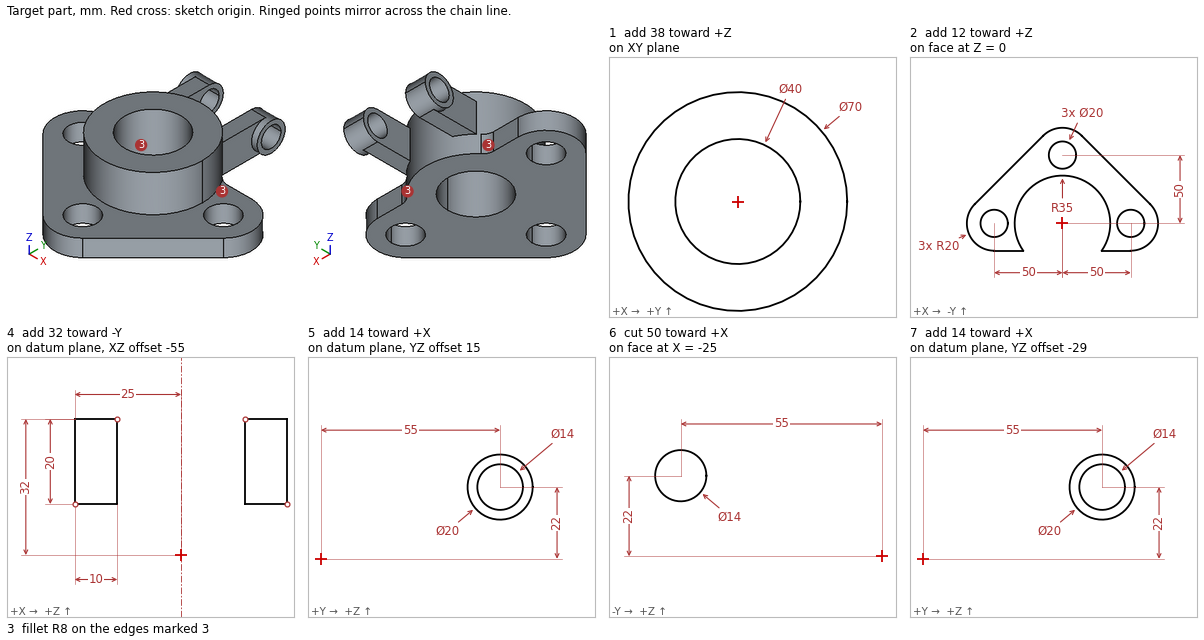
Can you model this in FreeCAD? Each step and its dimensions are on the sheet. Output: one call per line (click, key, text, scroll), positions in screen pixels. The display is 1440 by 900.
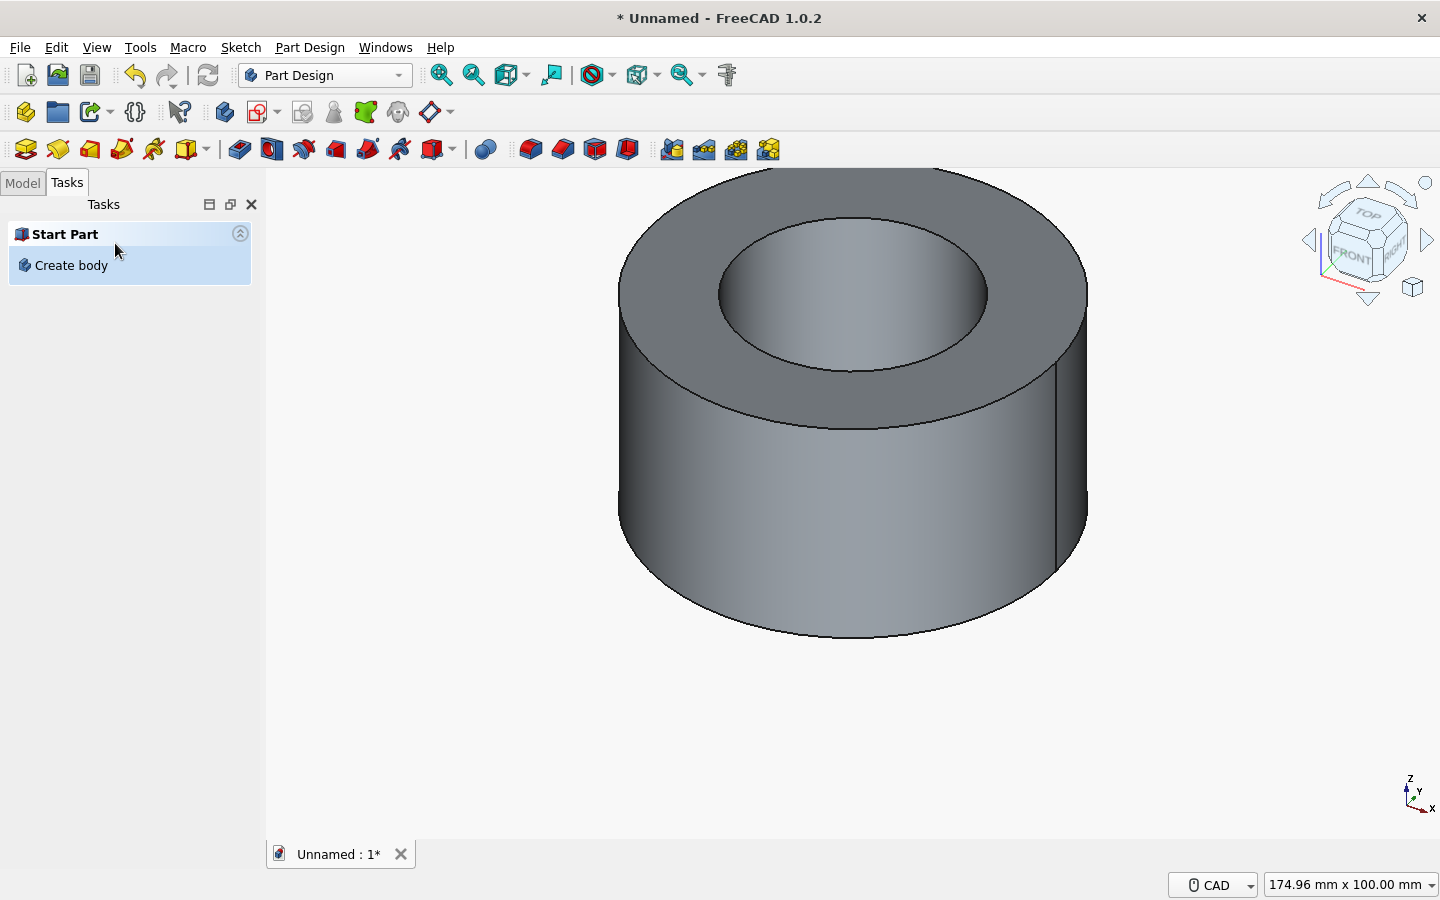
click(442, 76)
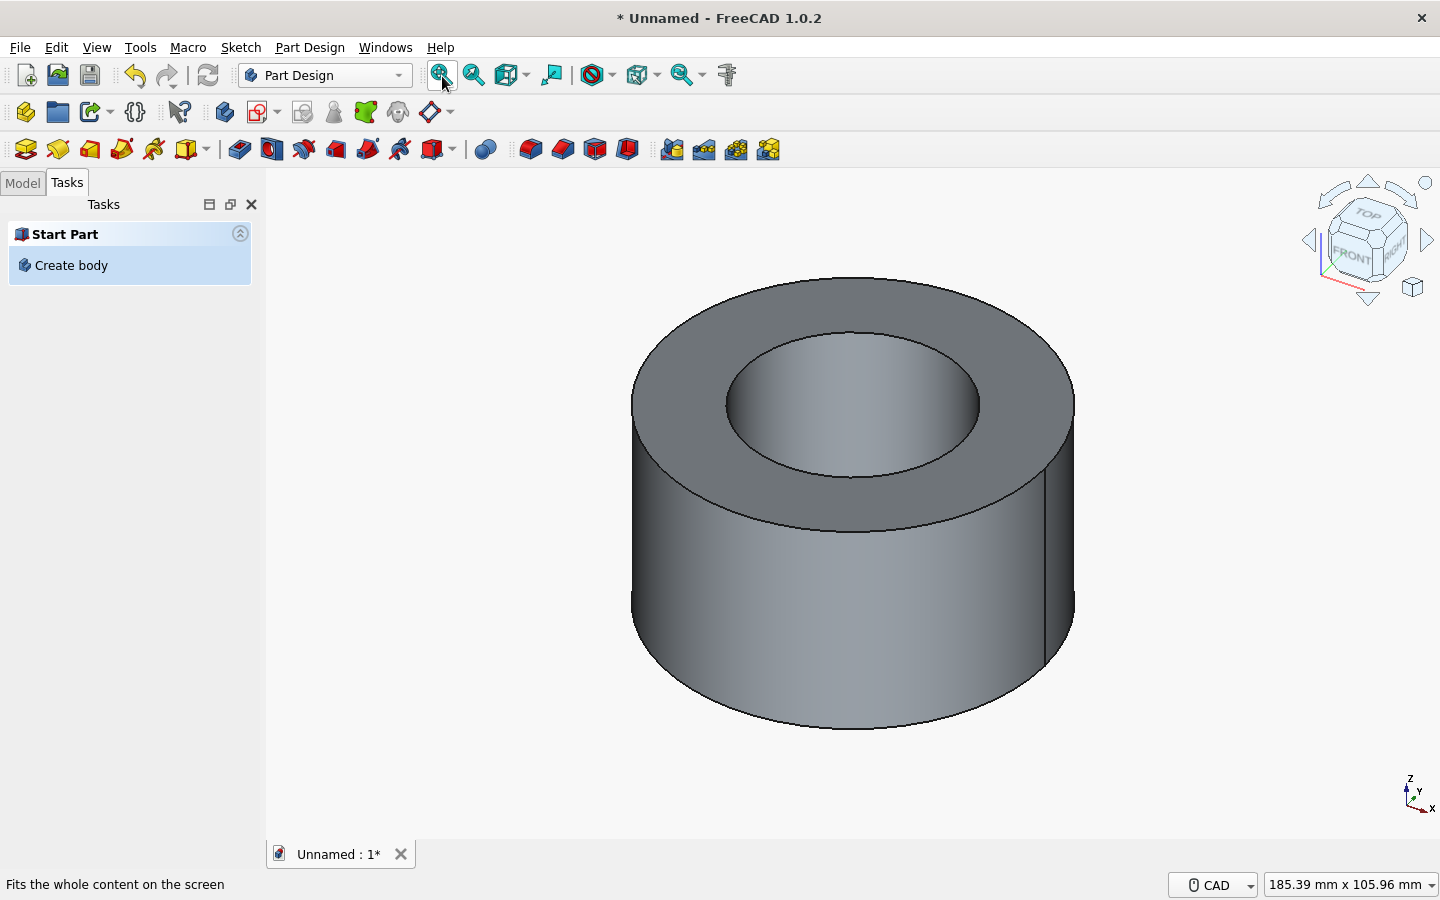
key(5)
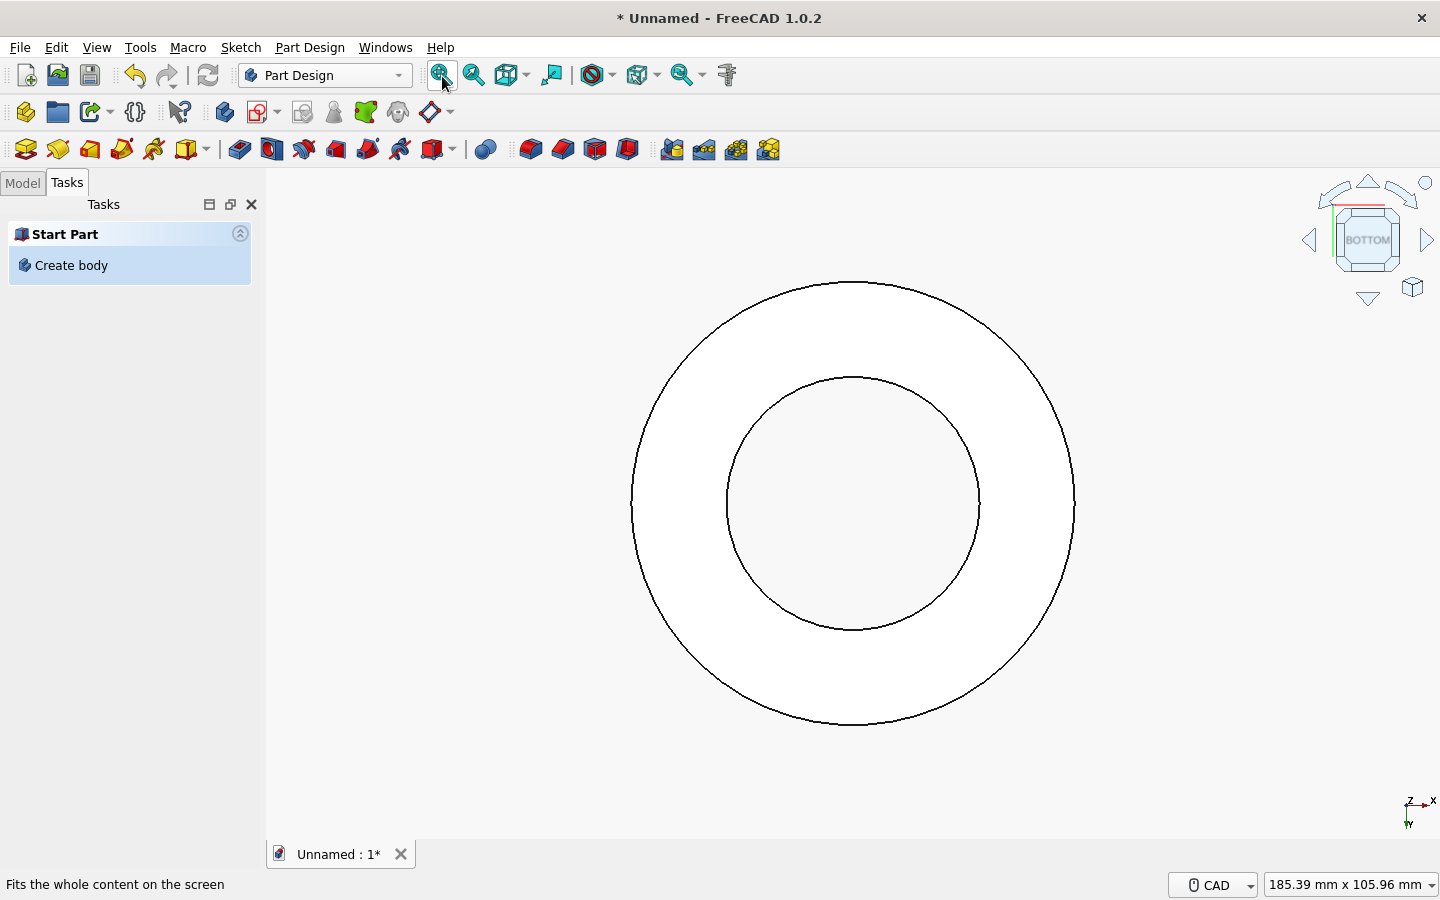
click(726, 376)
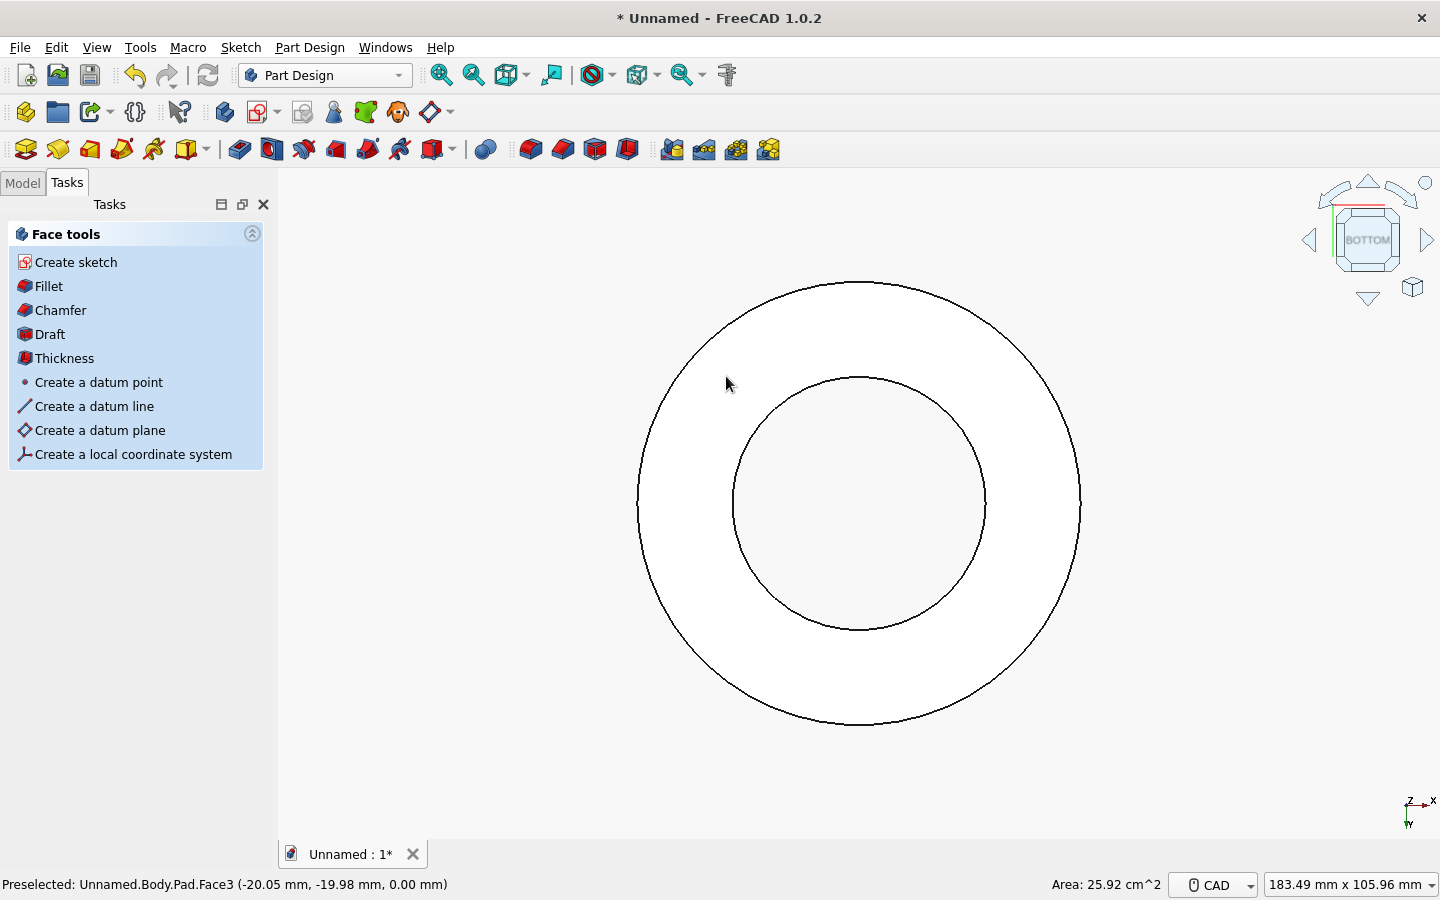
click(258, 112)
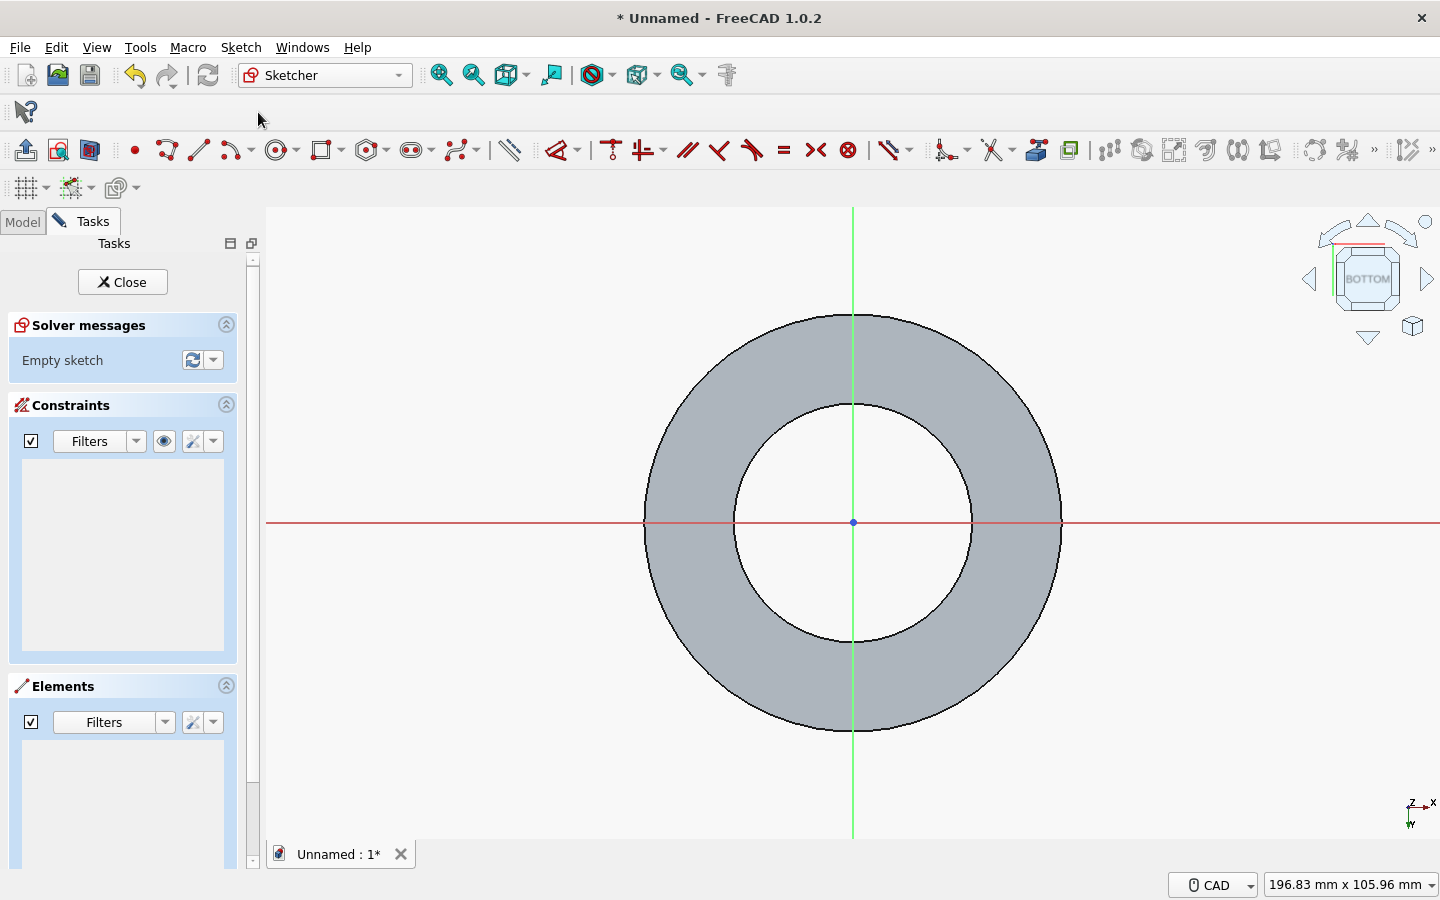
scroll(645, 811, down, 2)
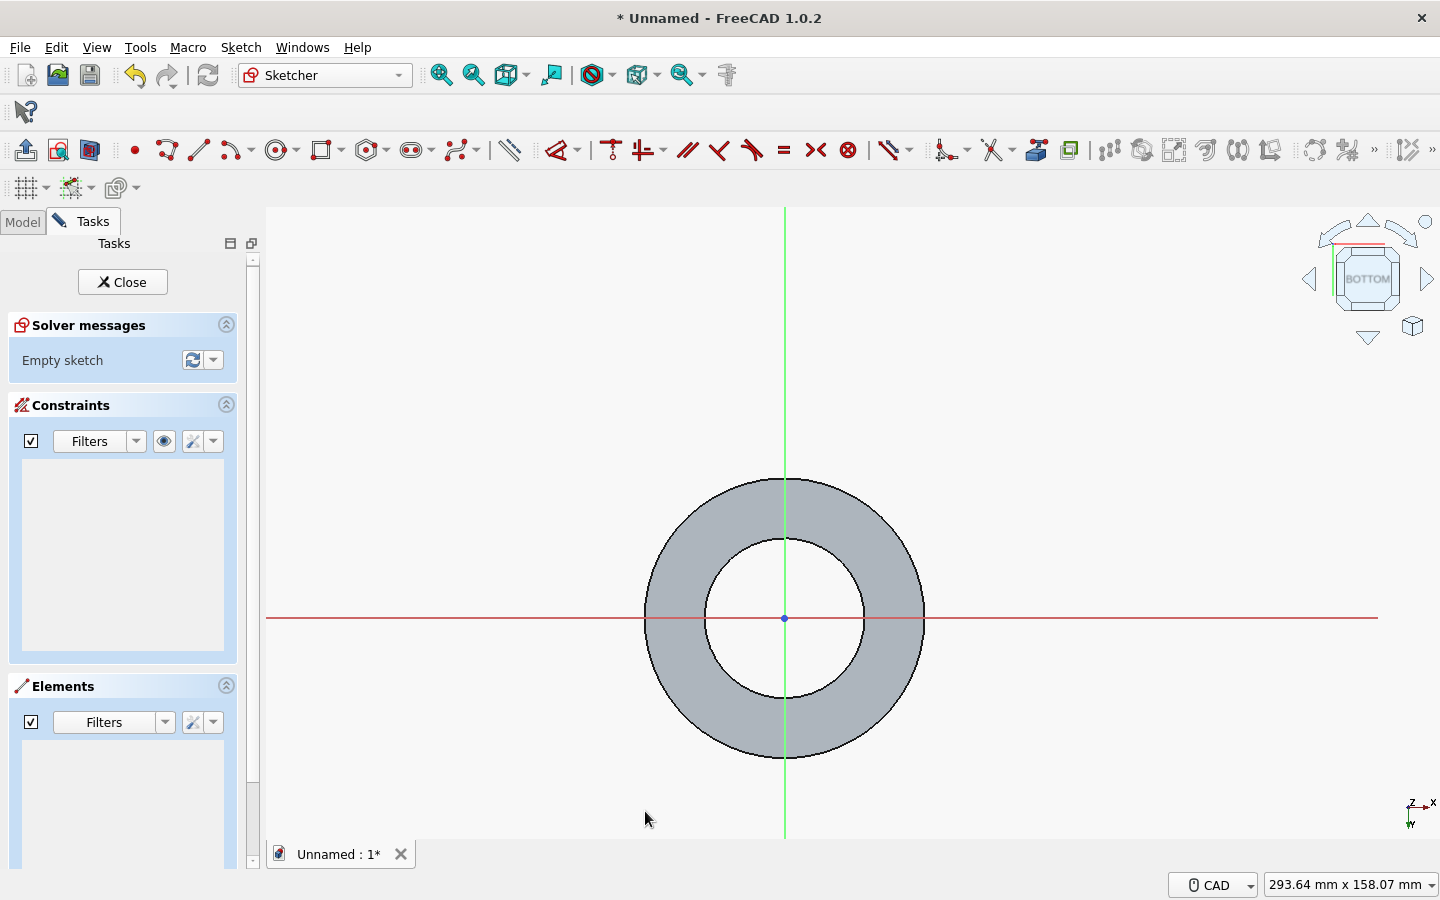
key(g)
key(l)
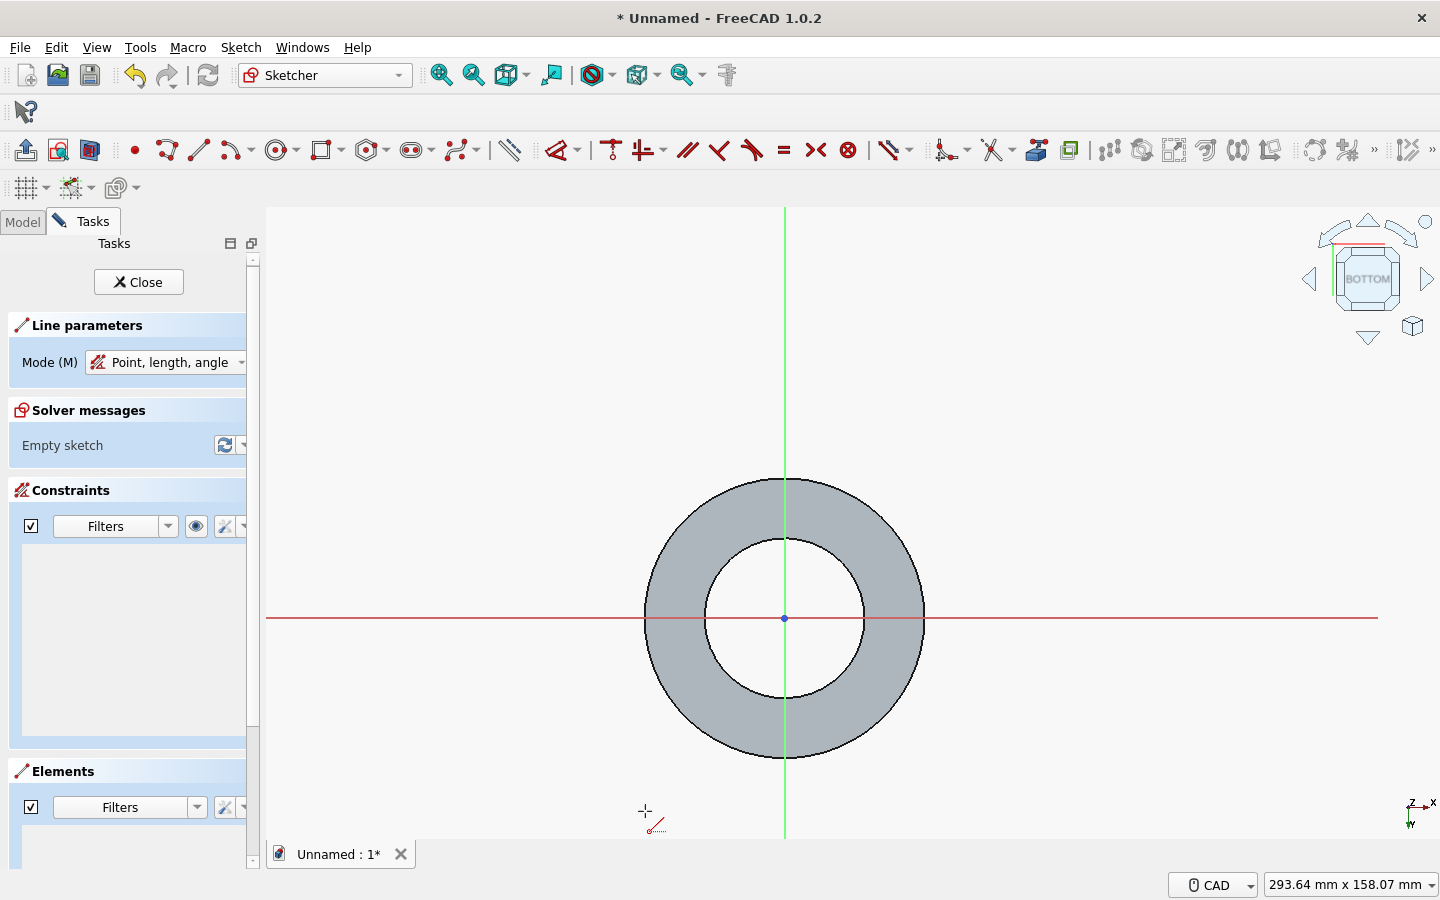
click(984, 698)
click(899, 698)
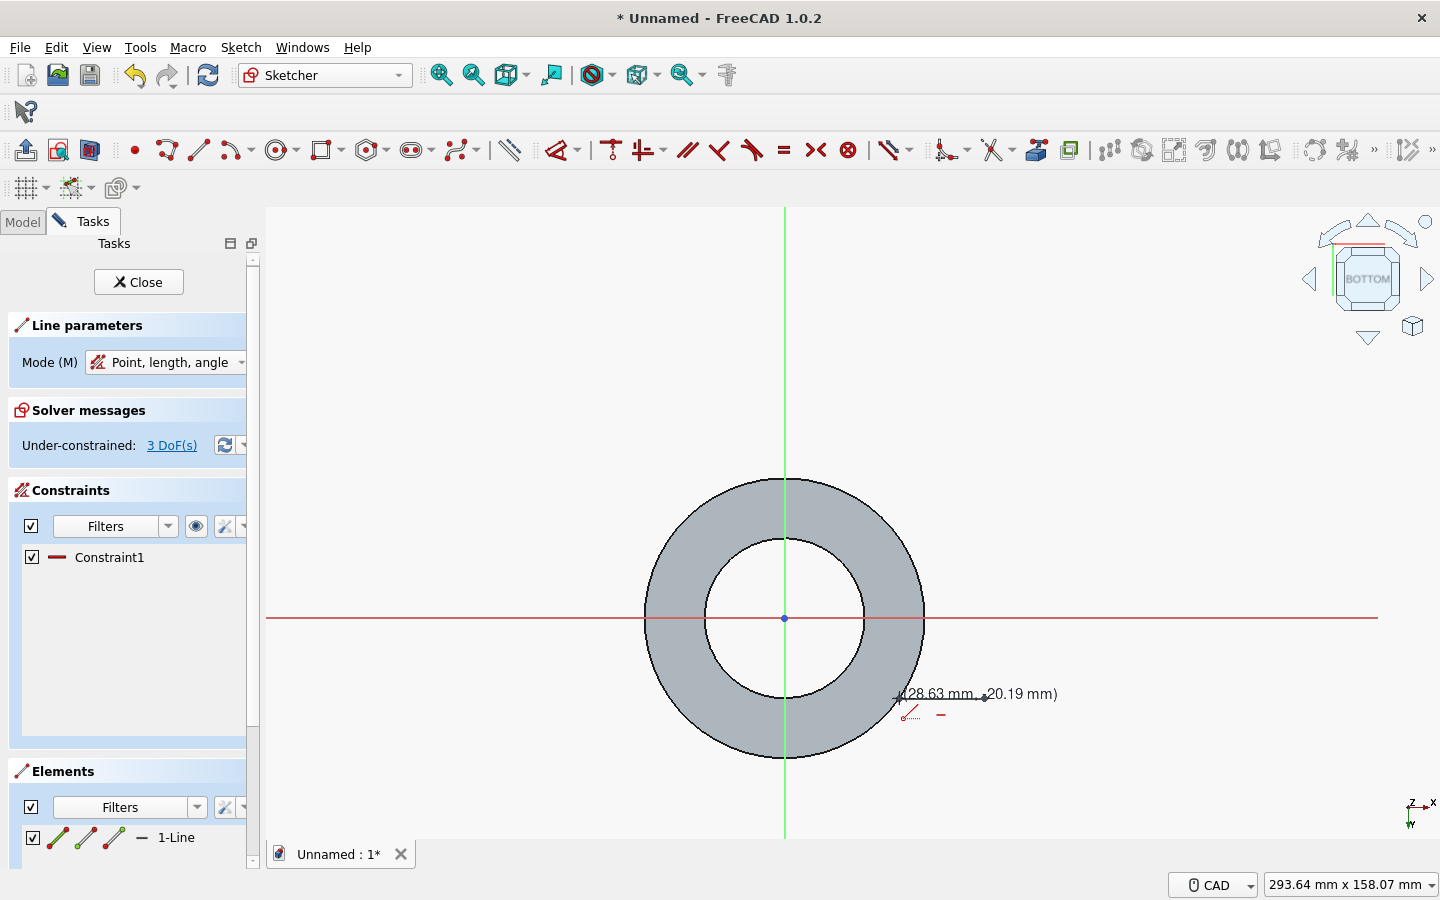
click(670, 698)
click(585, 698)